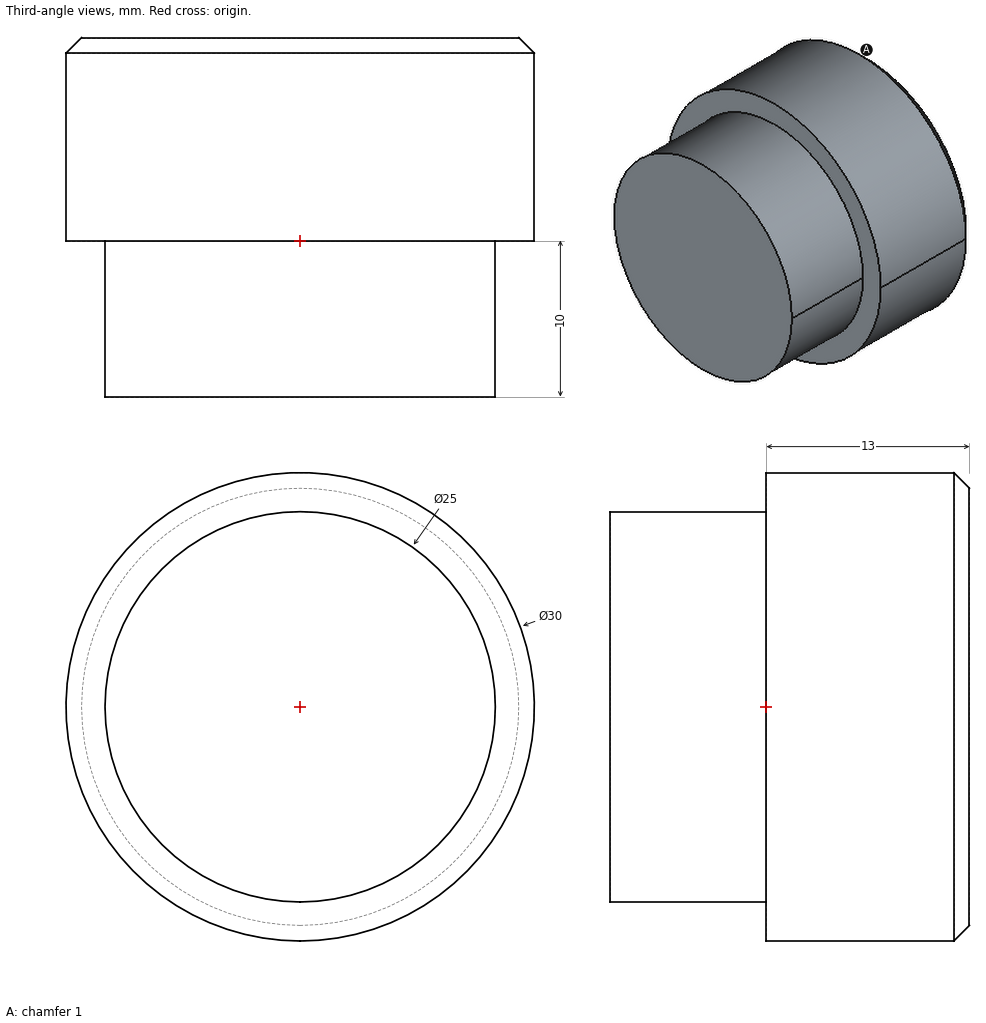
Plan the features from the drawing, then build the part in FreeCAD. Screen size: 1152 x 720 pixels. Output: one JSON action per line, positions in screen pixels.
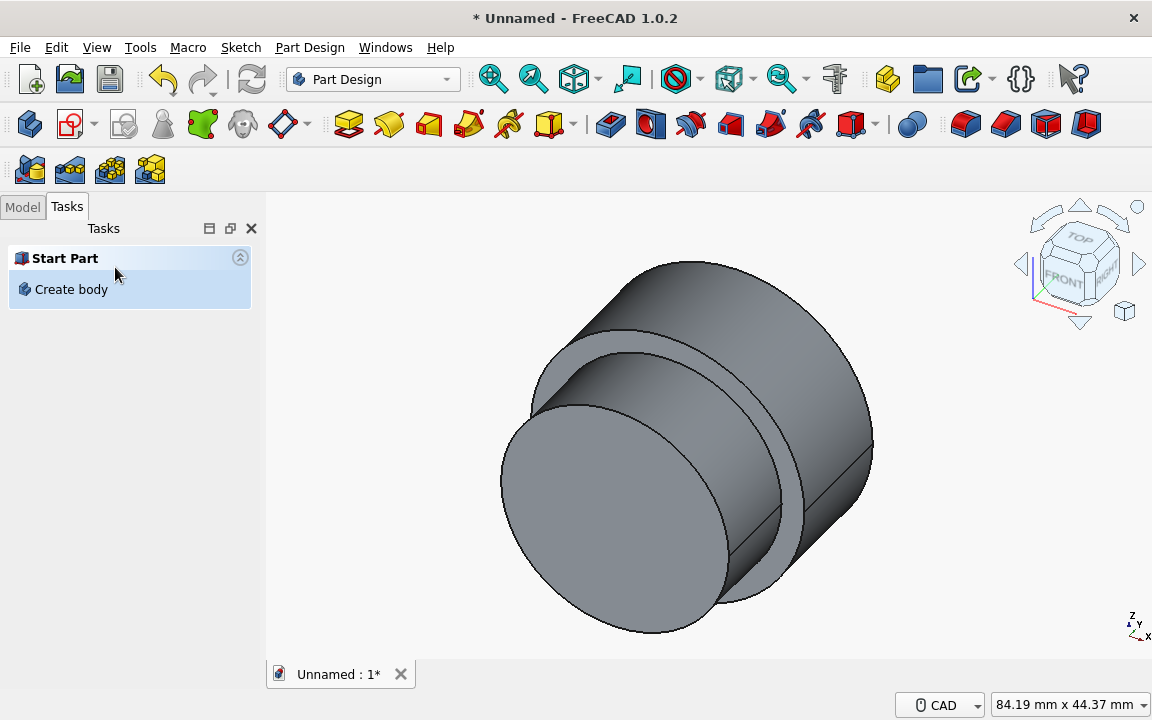
{"action": "left_click", "coordinate": [494, 80]}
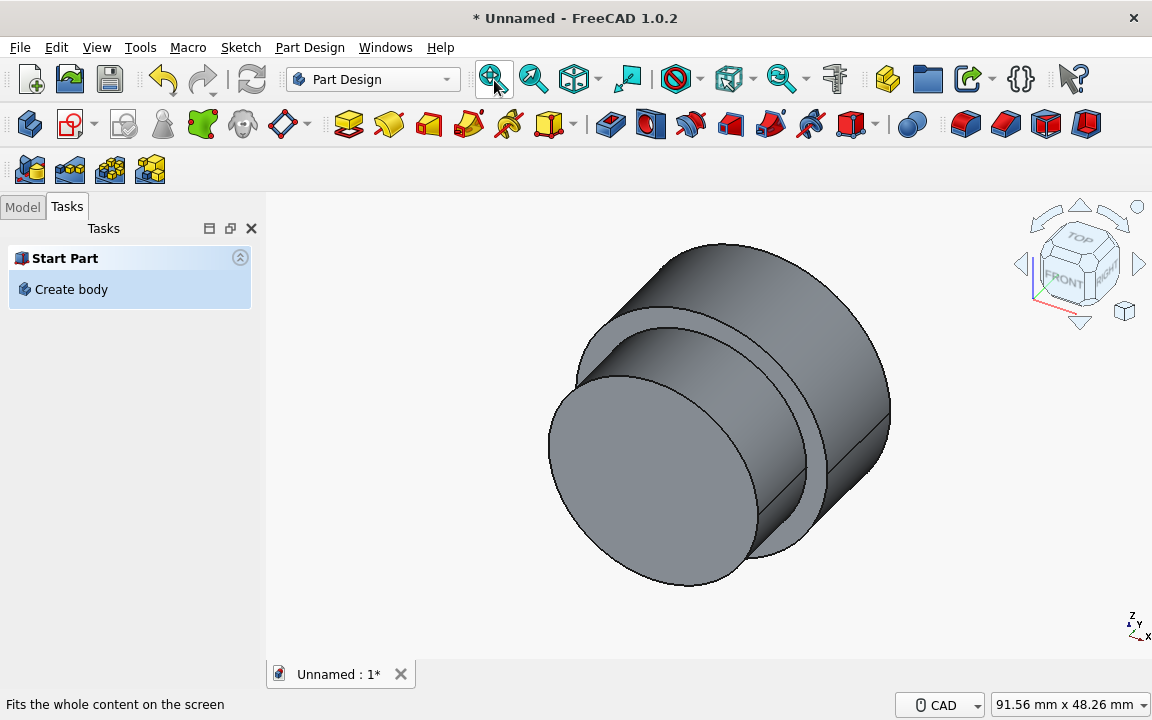
{"action": "key", "text": "0"}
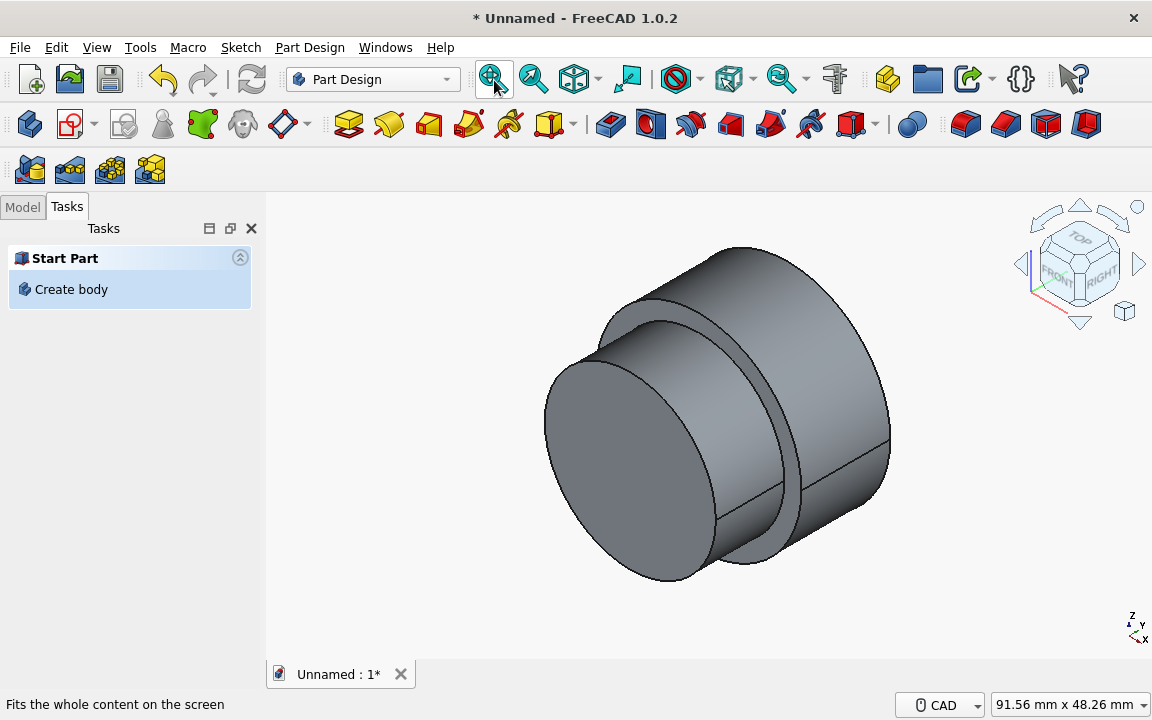
{"action": "key", "text": "2"}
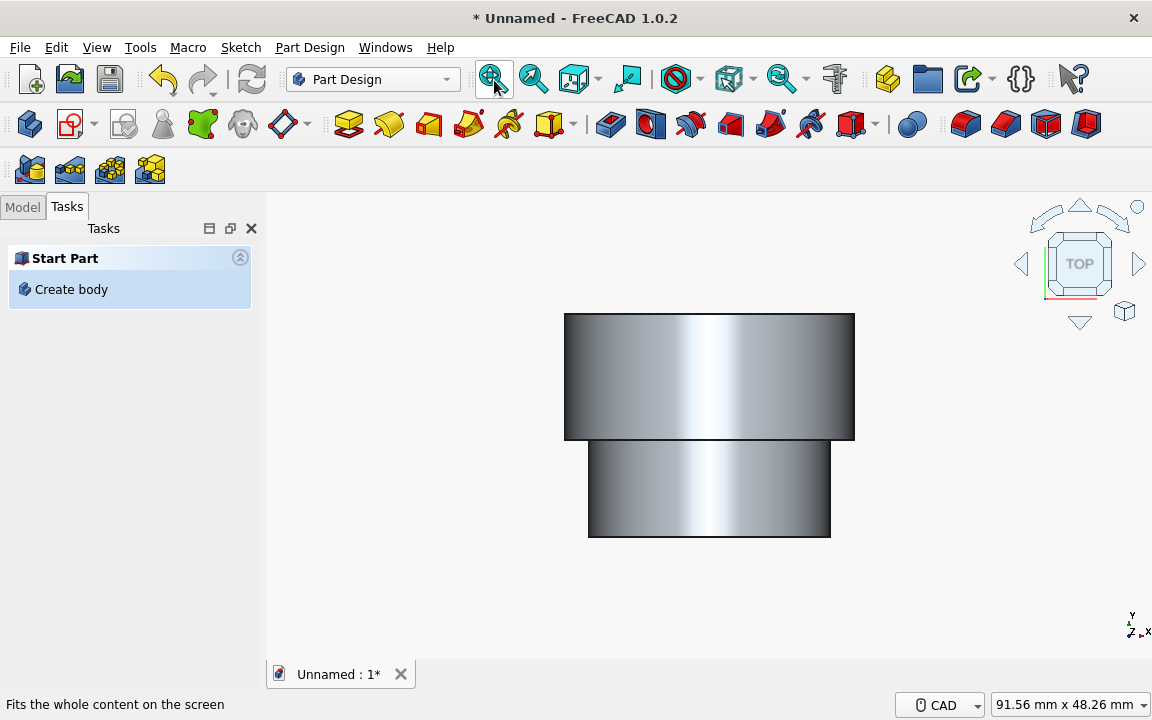
{"action": "left_click", "coordinate": [592, 313]}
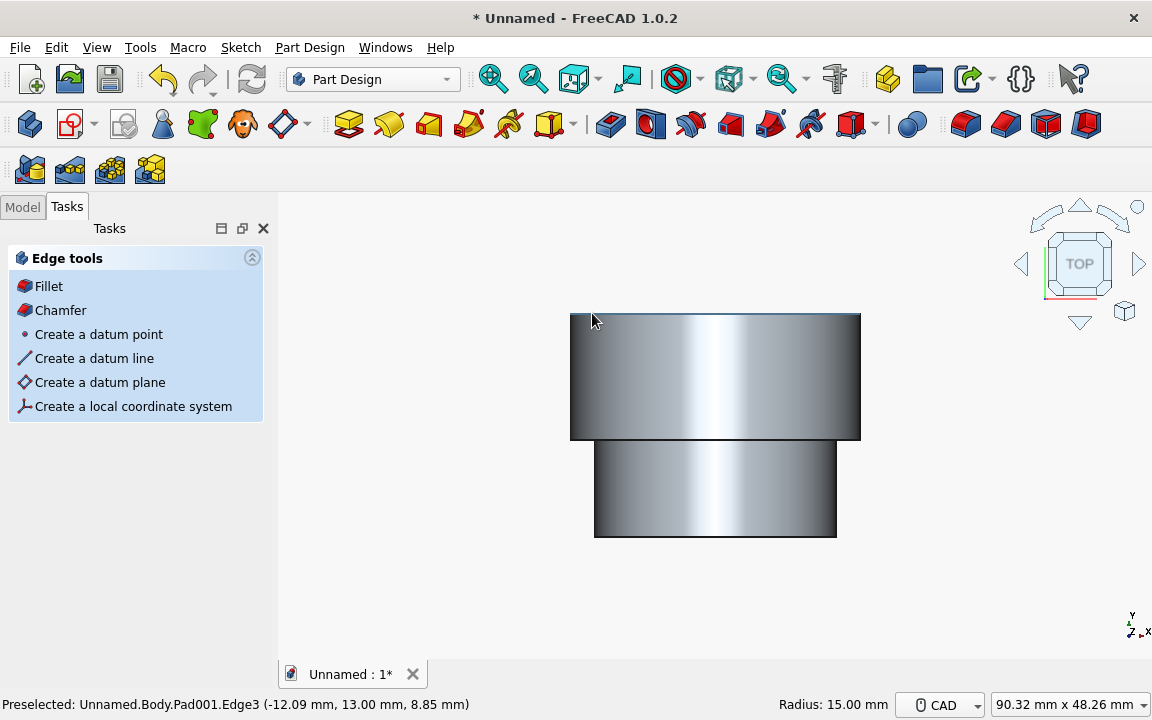
{"action": "left_click", "coordinate": [1006, 124]}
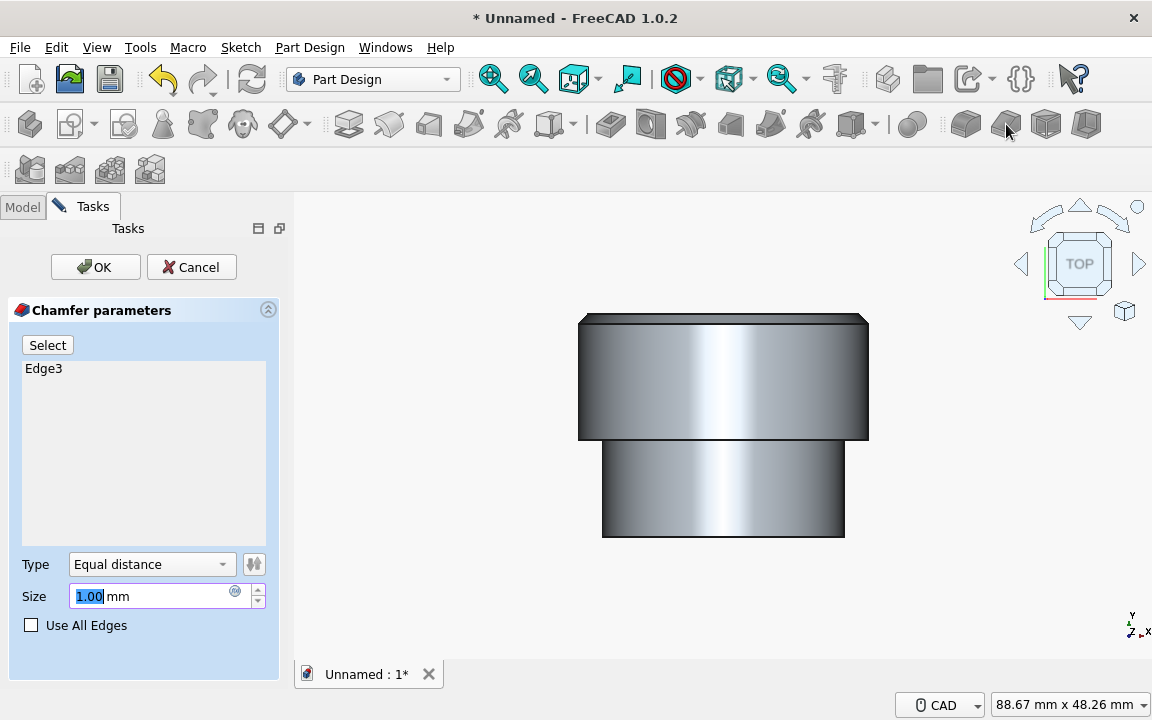
{"action": "type", "text": "1"}
{"action": "key", "text": "Tab"}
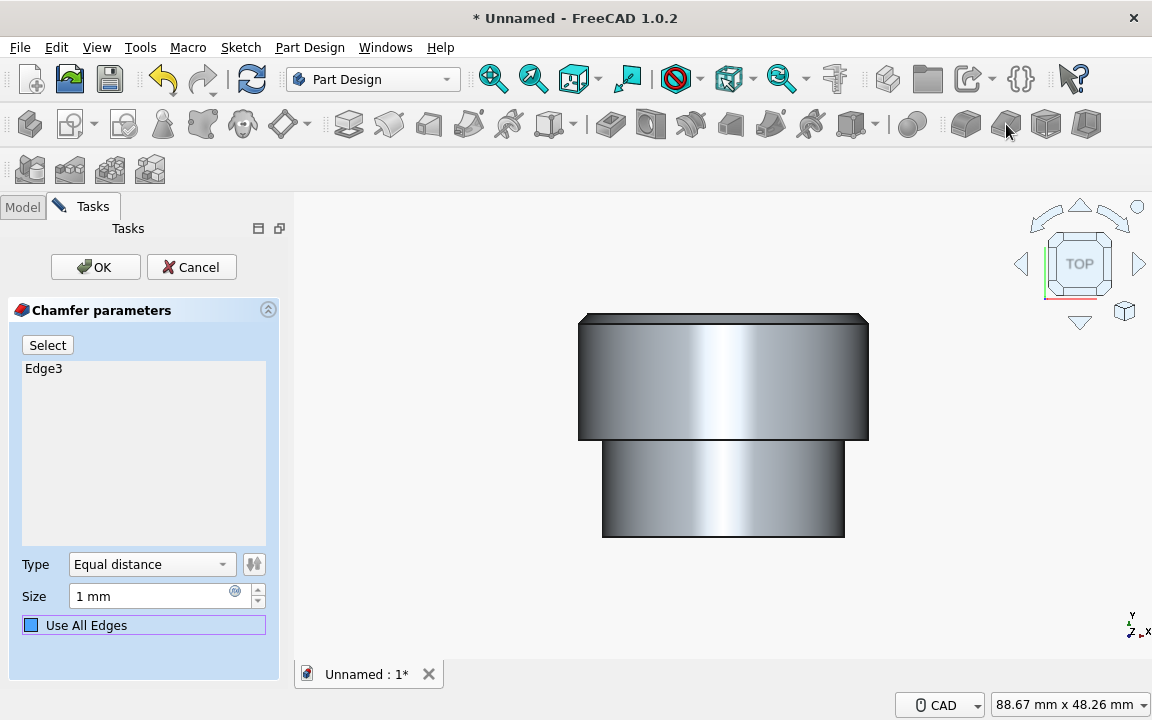
{"action": "left_click", "coordinate": [96, 267]}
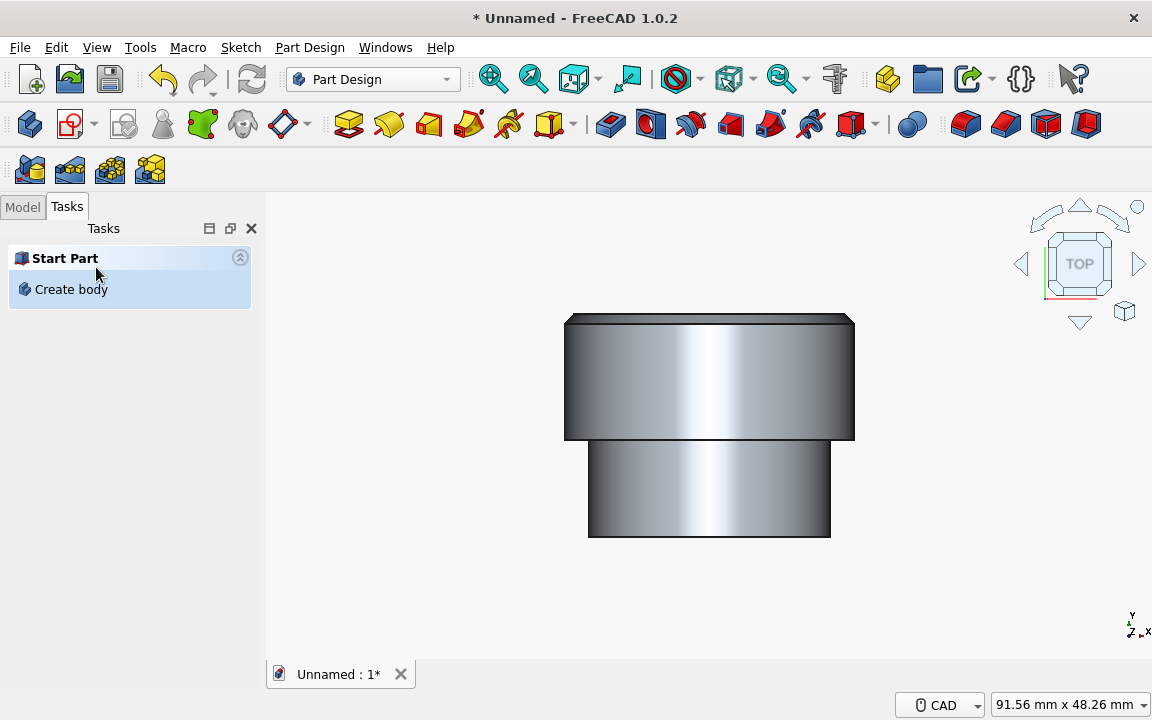
{"action": "key", "text": "0"}